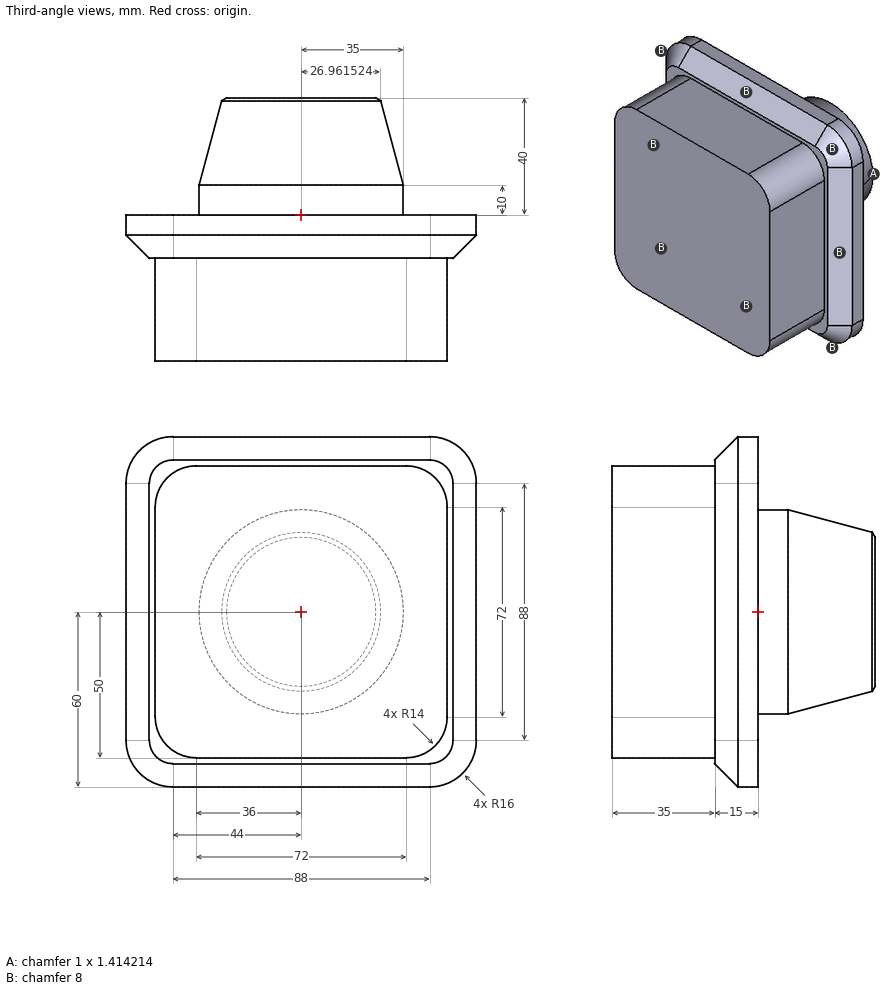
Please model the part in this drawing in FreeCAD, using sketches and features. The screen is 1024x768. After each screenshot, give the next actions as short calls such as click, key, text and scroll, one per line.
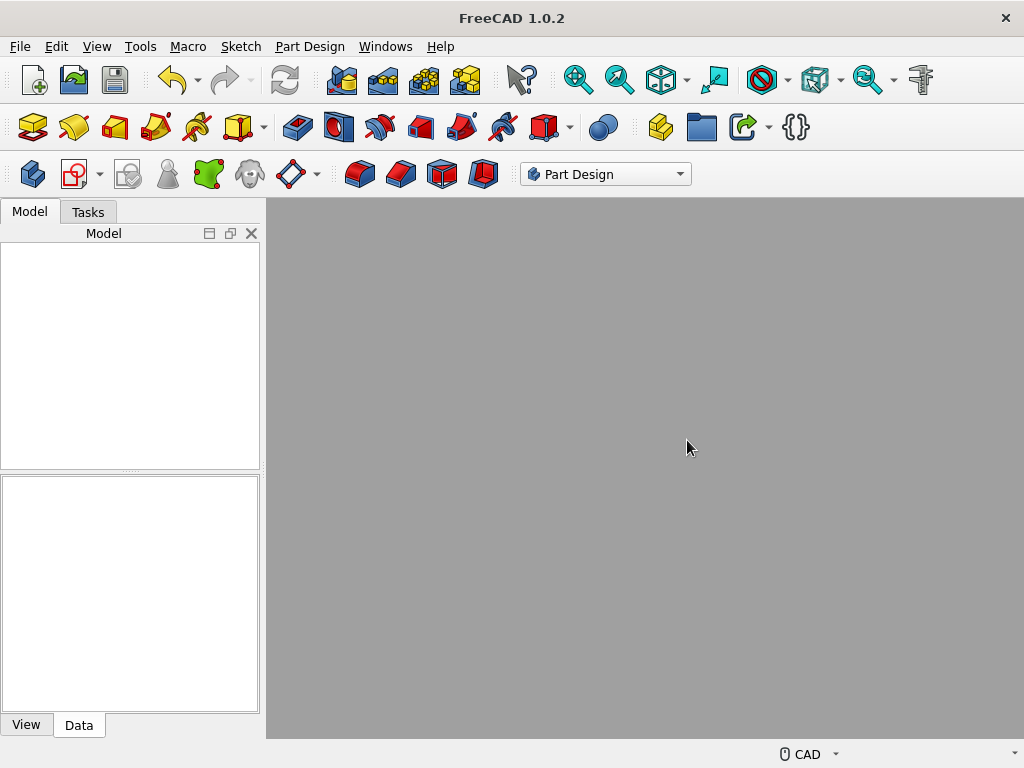
click(33, 80)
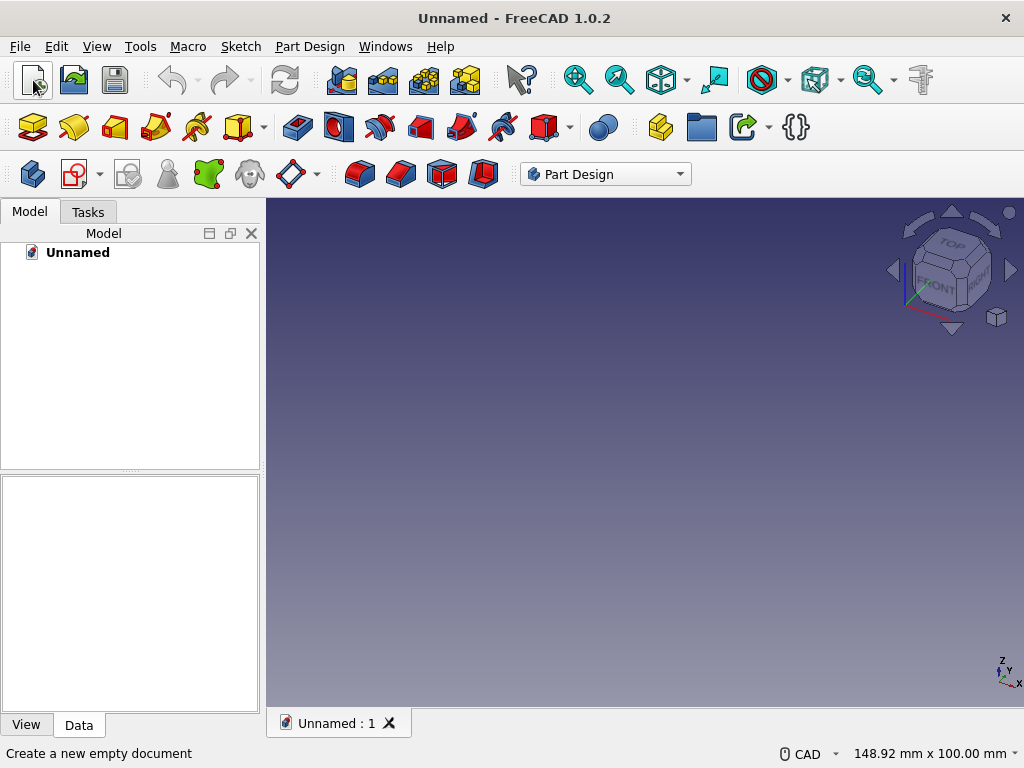
click(74, 174)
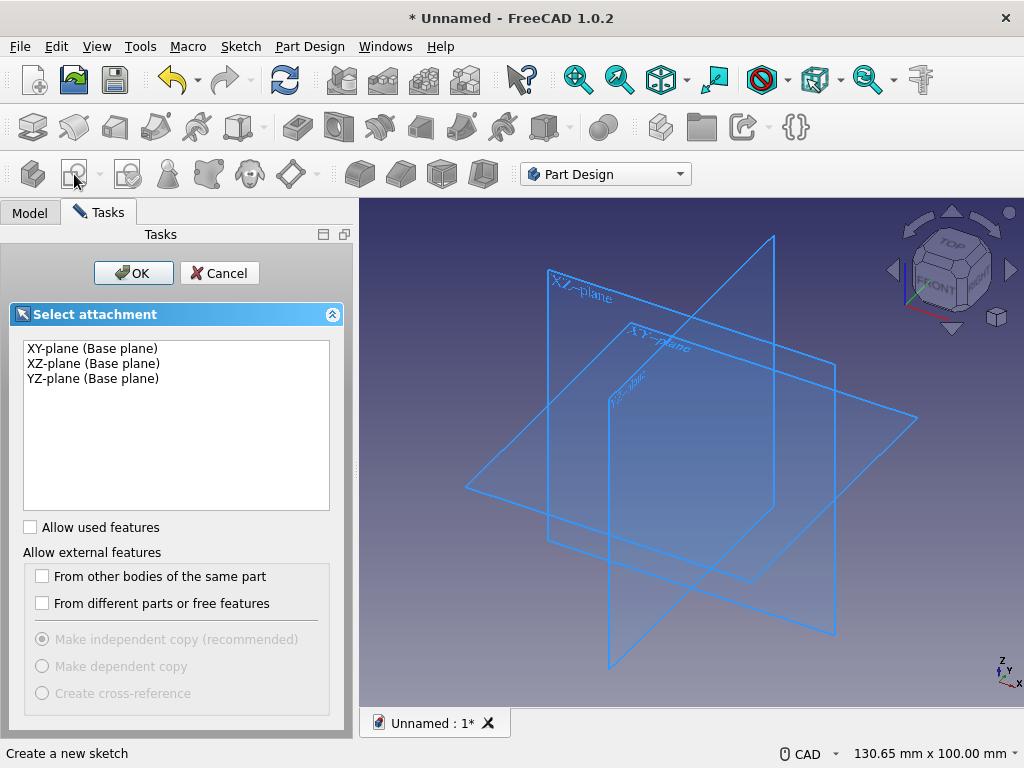
click(84, 348)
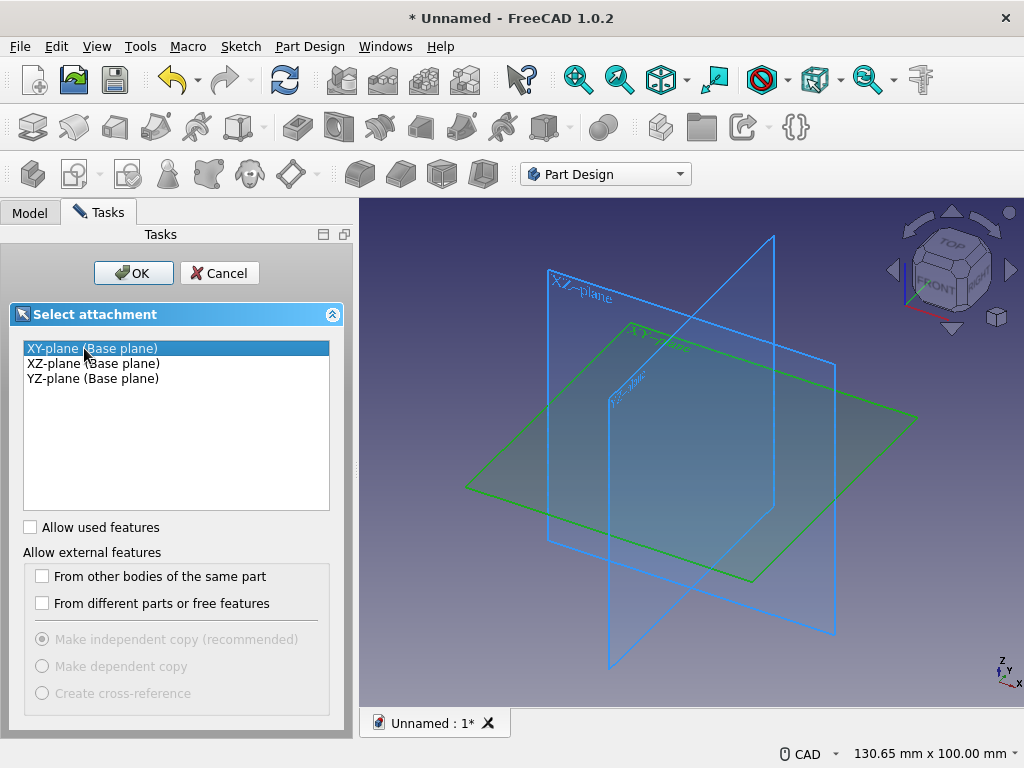
click(134, 273)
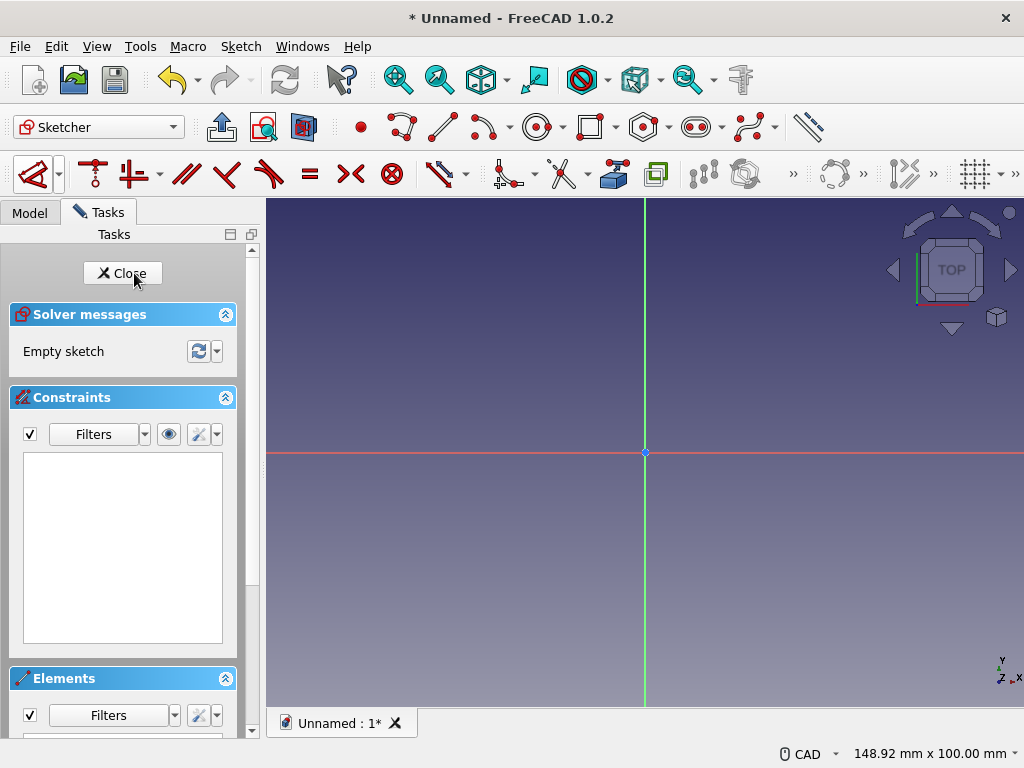
scroll(859, 226, up, 2)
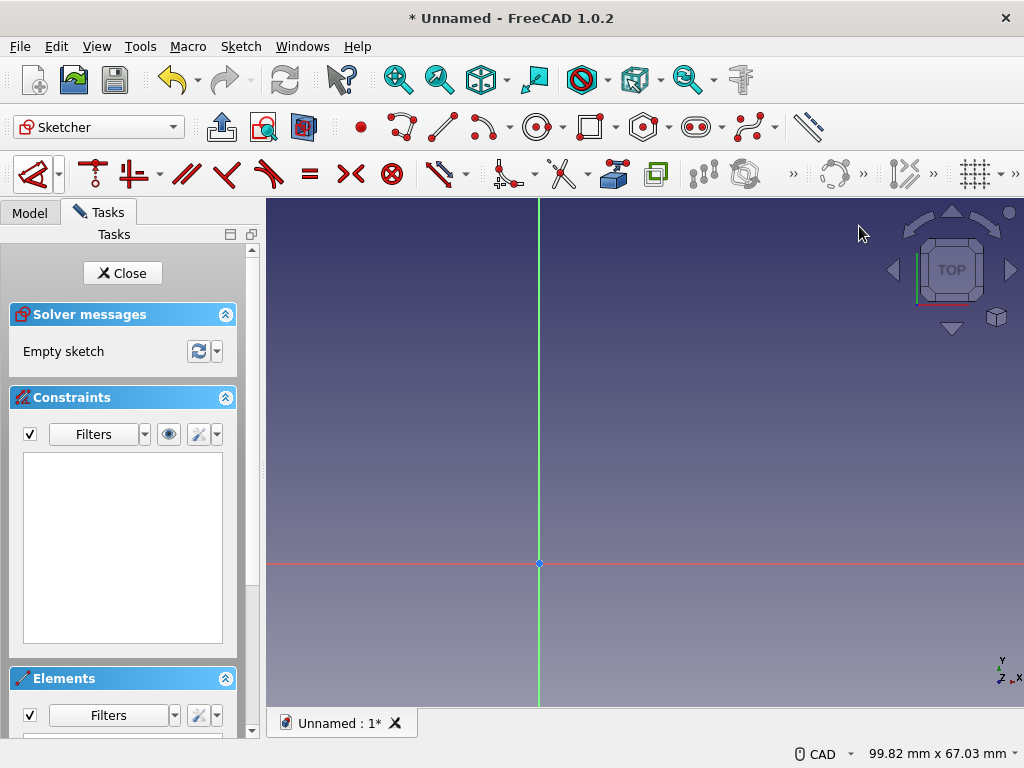
key(g)
key(m)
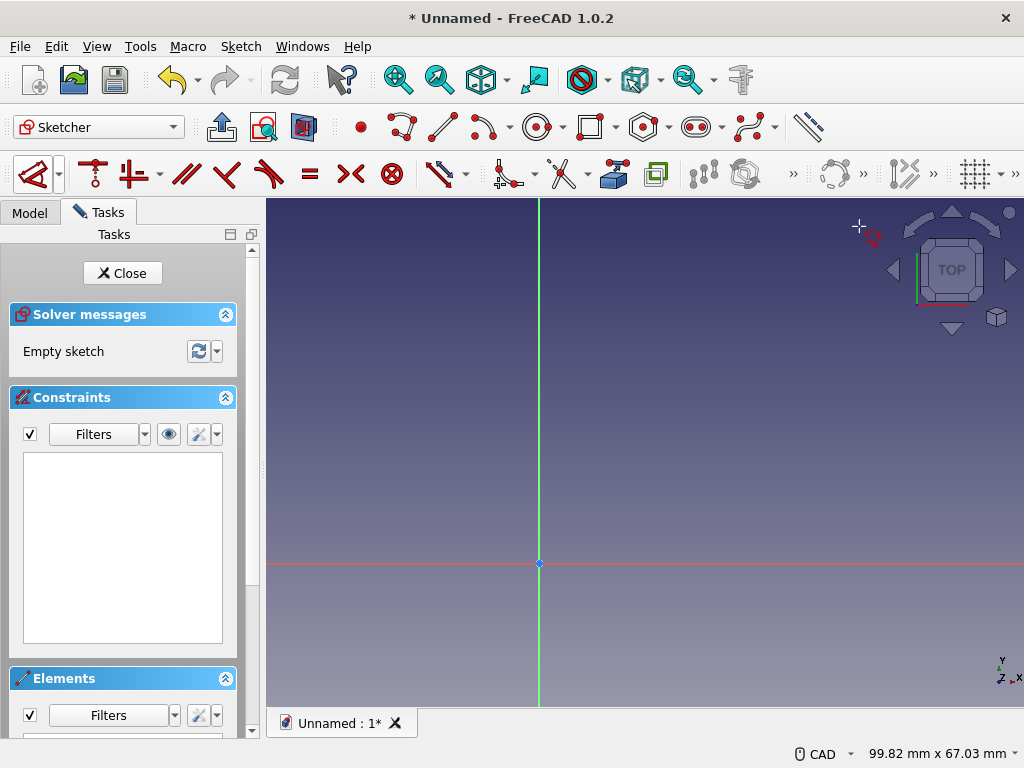
click(539, 564)
click(805, 555)
click(805, 488)
click(744, 260)
click(548, 260)
click(539, 564)
key(Escape)
key(Escape)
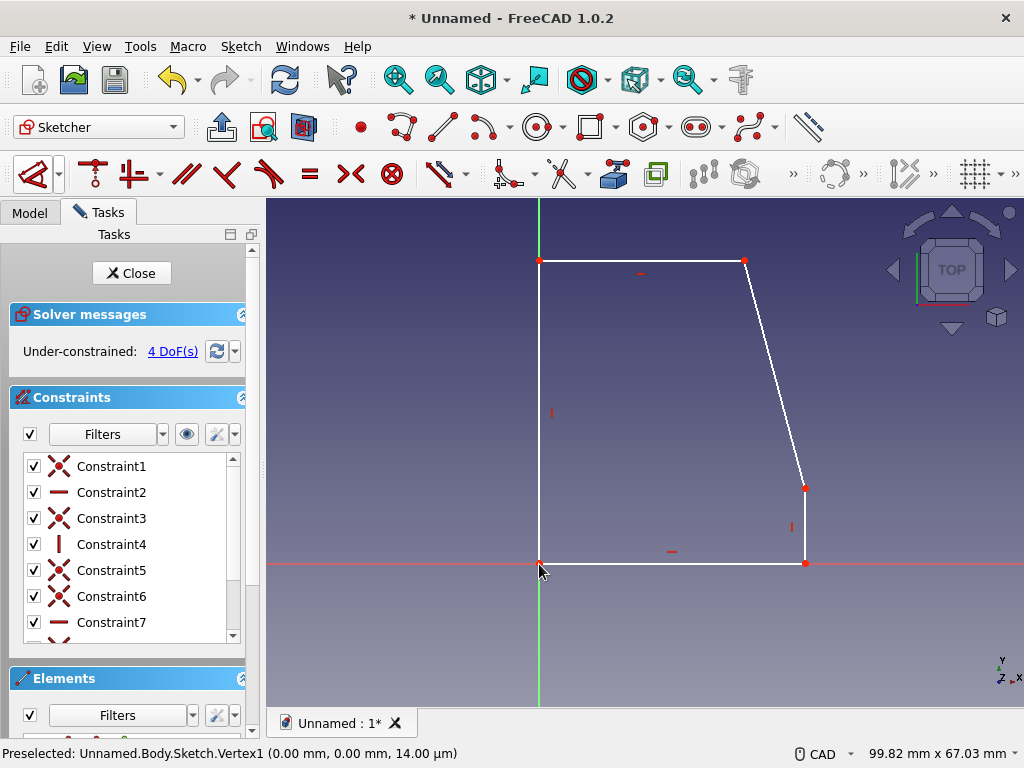
key(d)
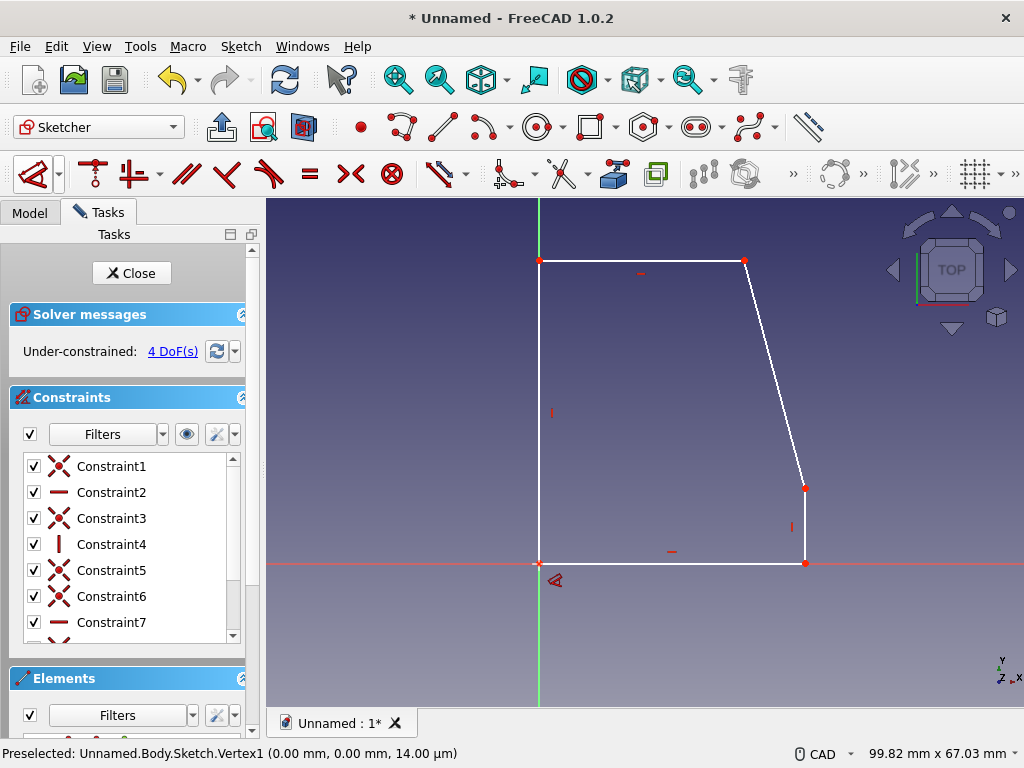
click(619, 564)
click(672, 598)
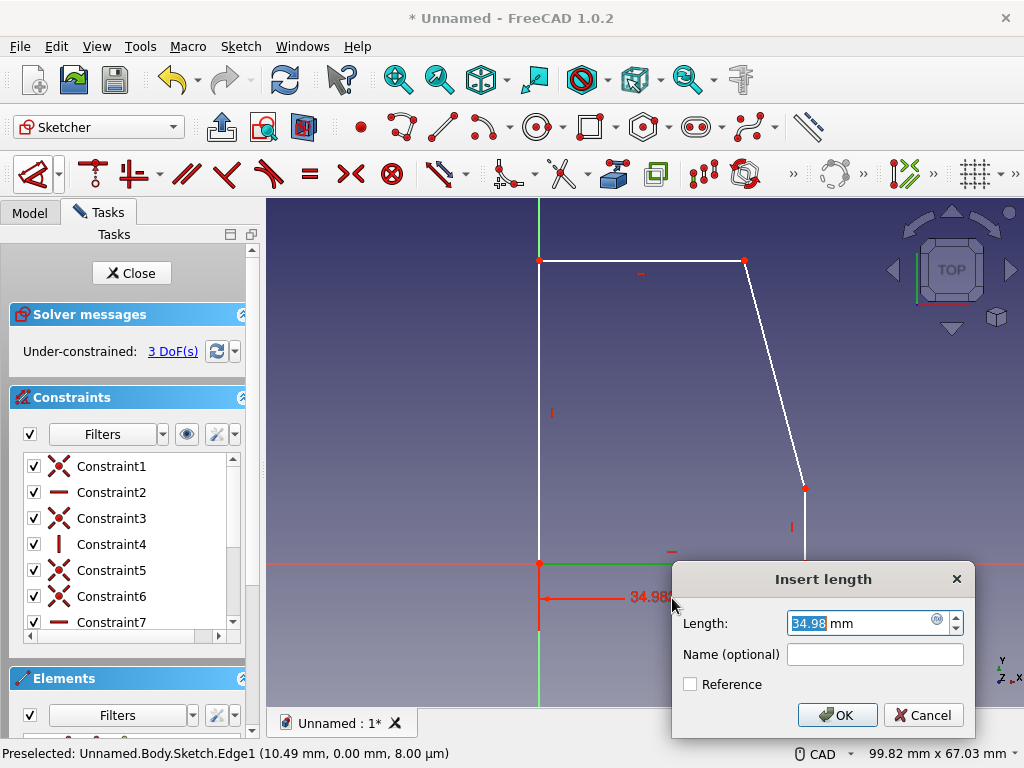
text(35)
key(Return)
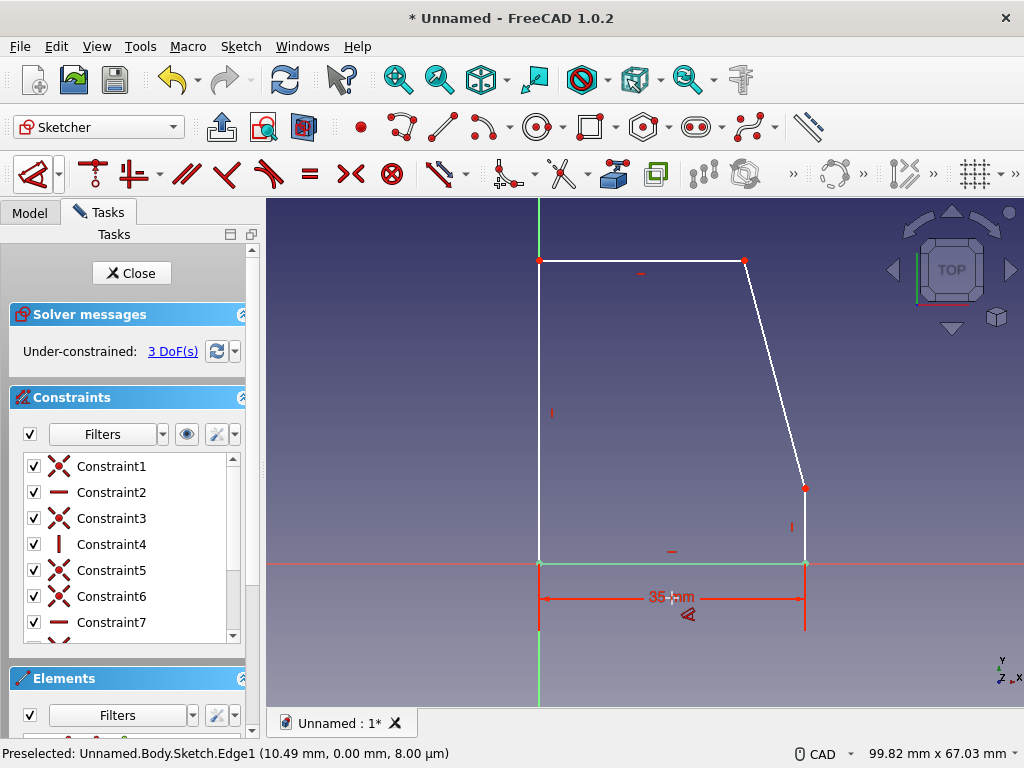
click(805, 541)
click(839, 526)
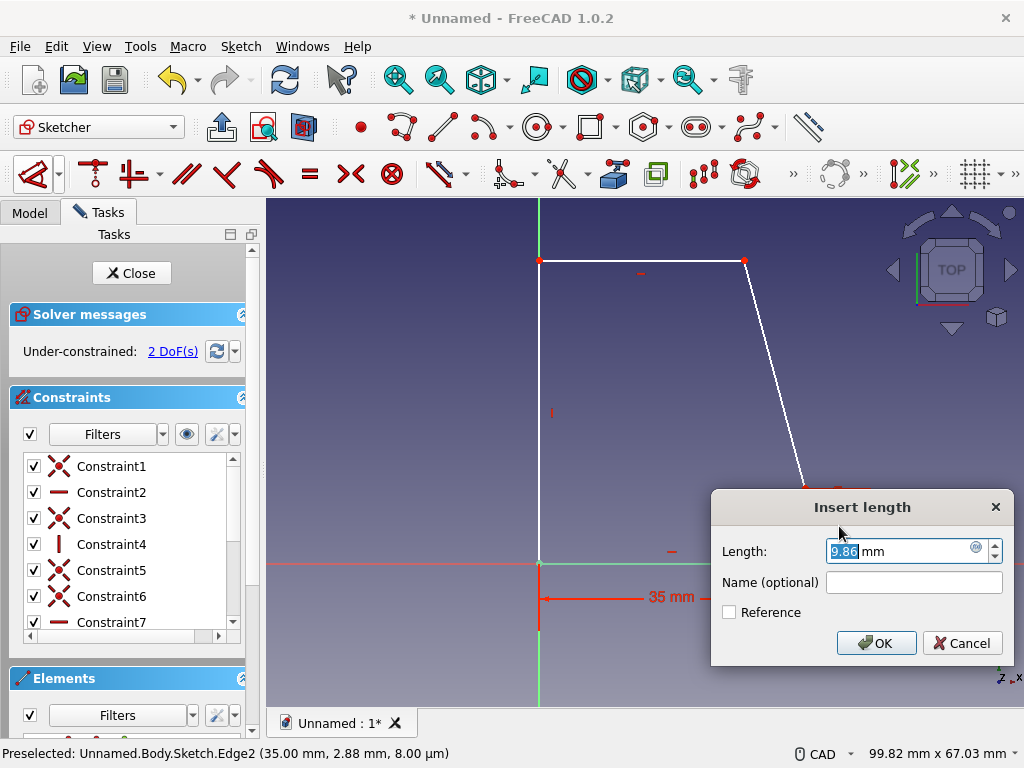
text(10)
key(Return)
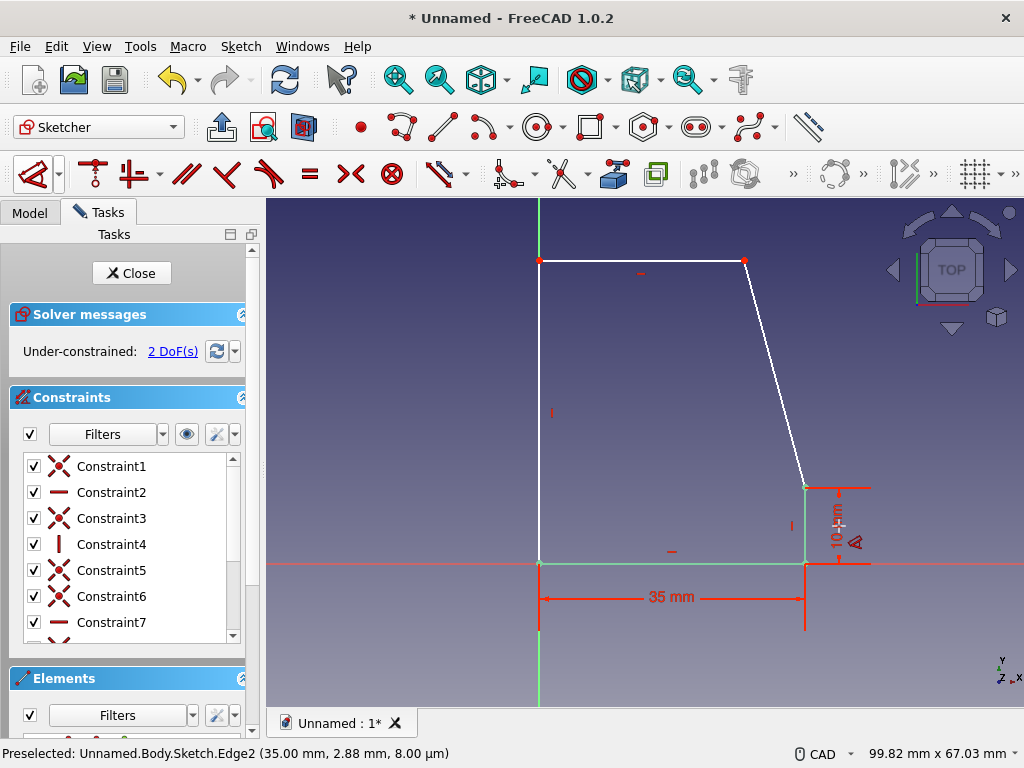
click(539, 352)
click(505, 412)